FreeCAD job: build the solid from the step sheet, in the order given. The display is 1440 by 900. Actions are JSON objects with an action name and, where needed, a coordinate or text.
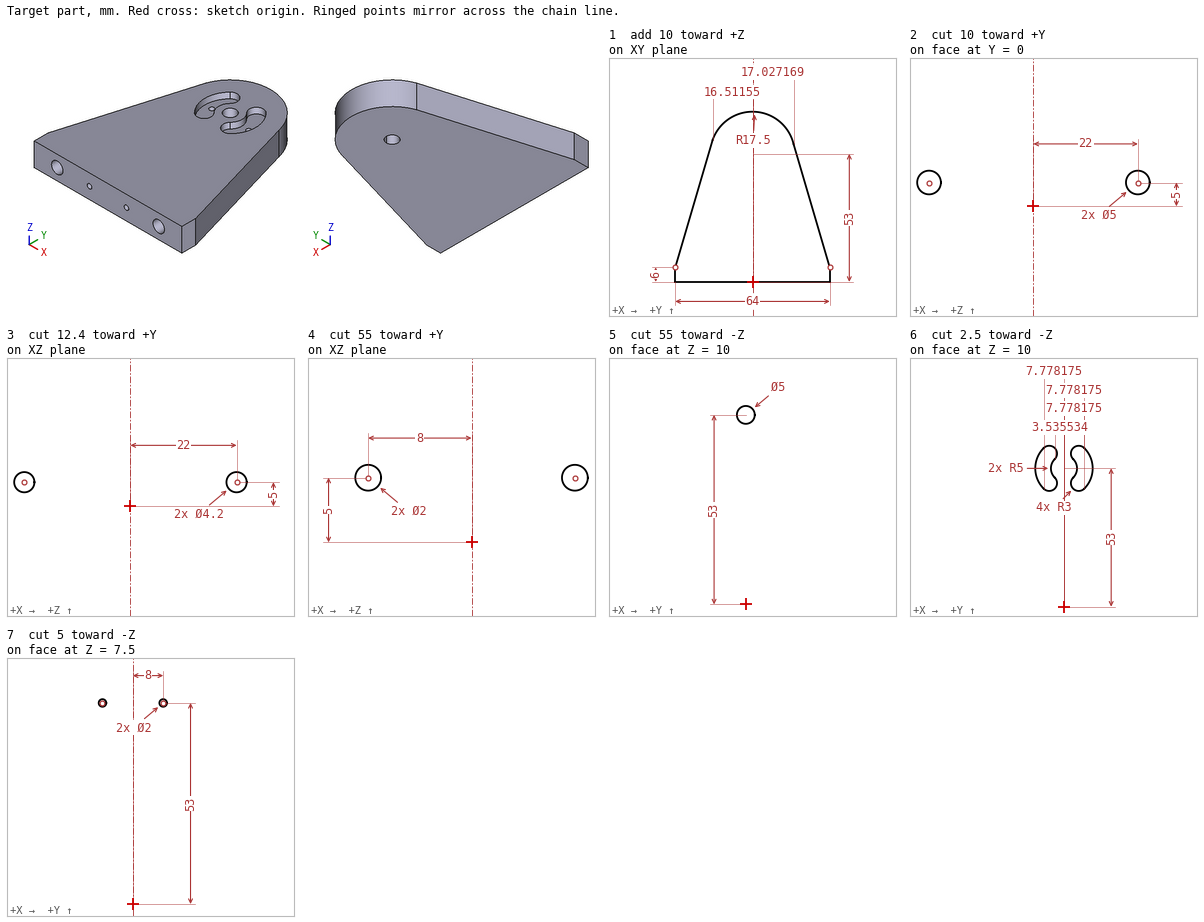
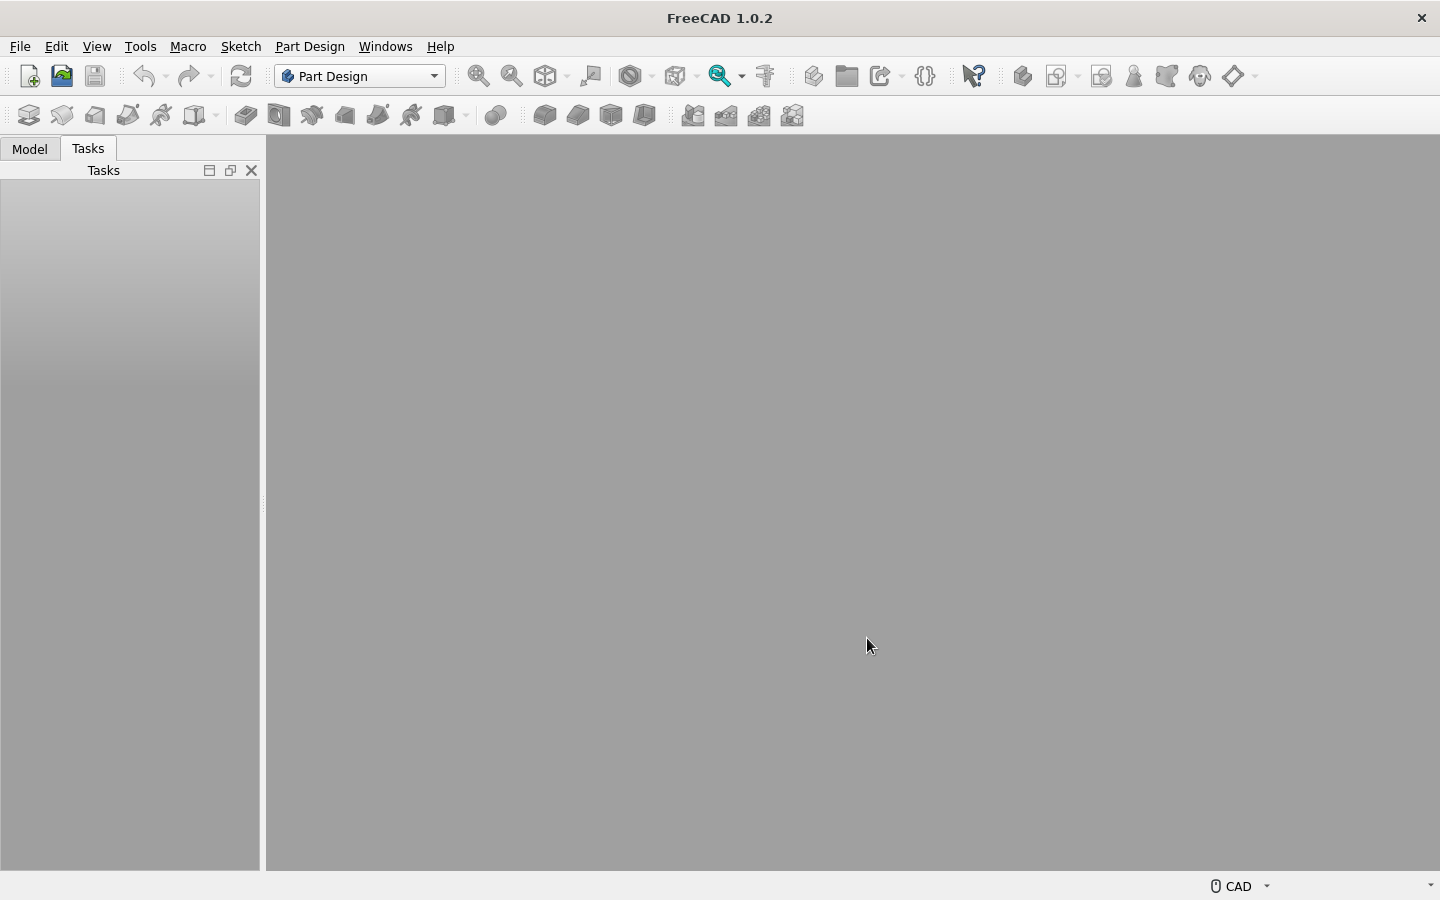
{"action": "left_click", "coordinate": [29, 76]}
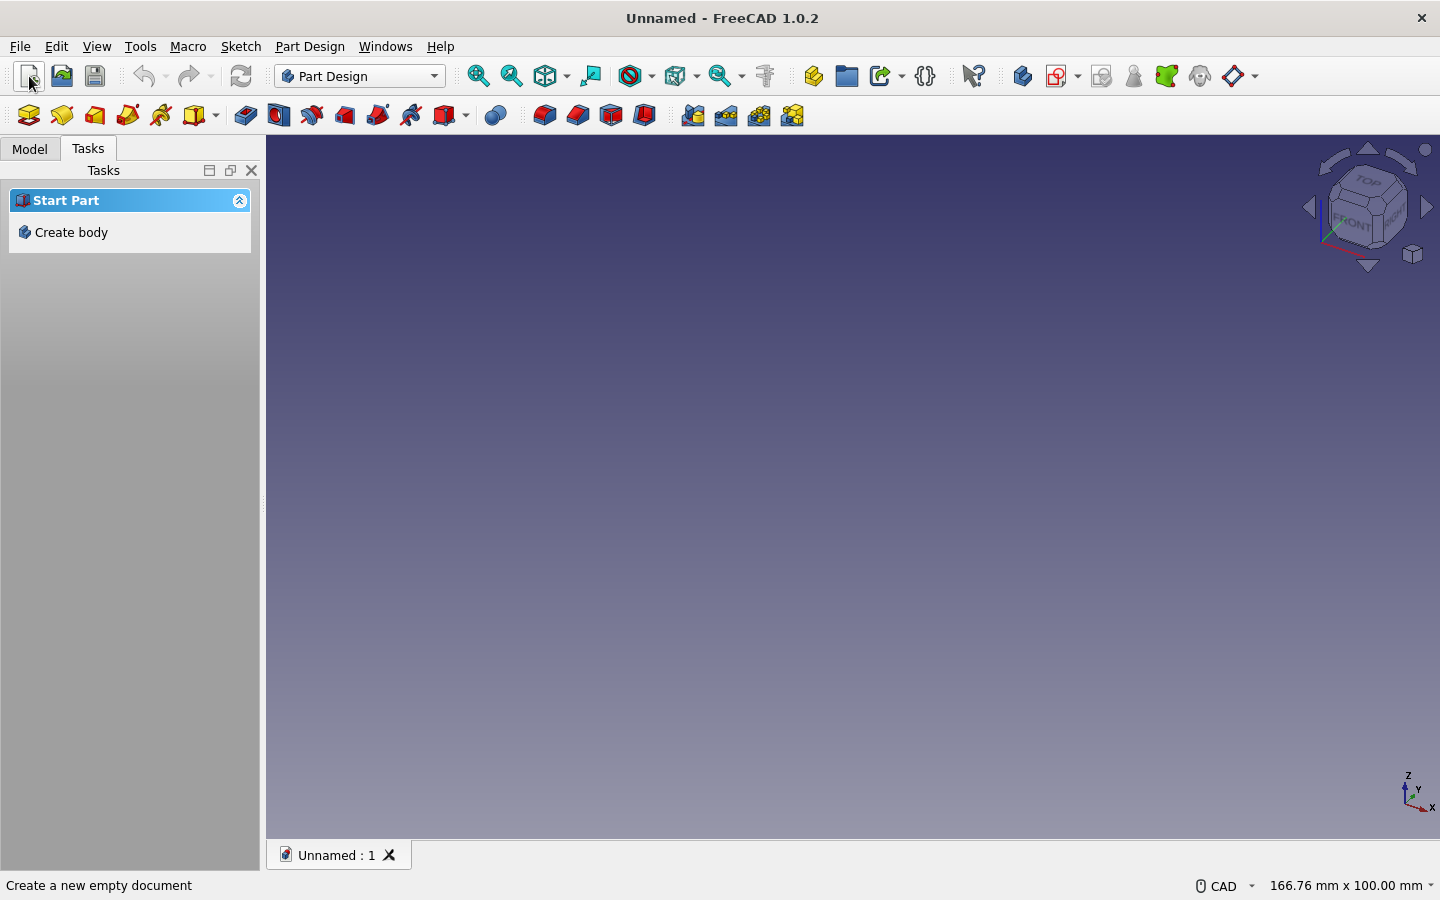
{"action": "left_click", "coordinate": [1056, 76]}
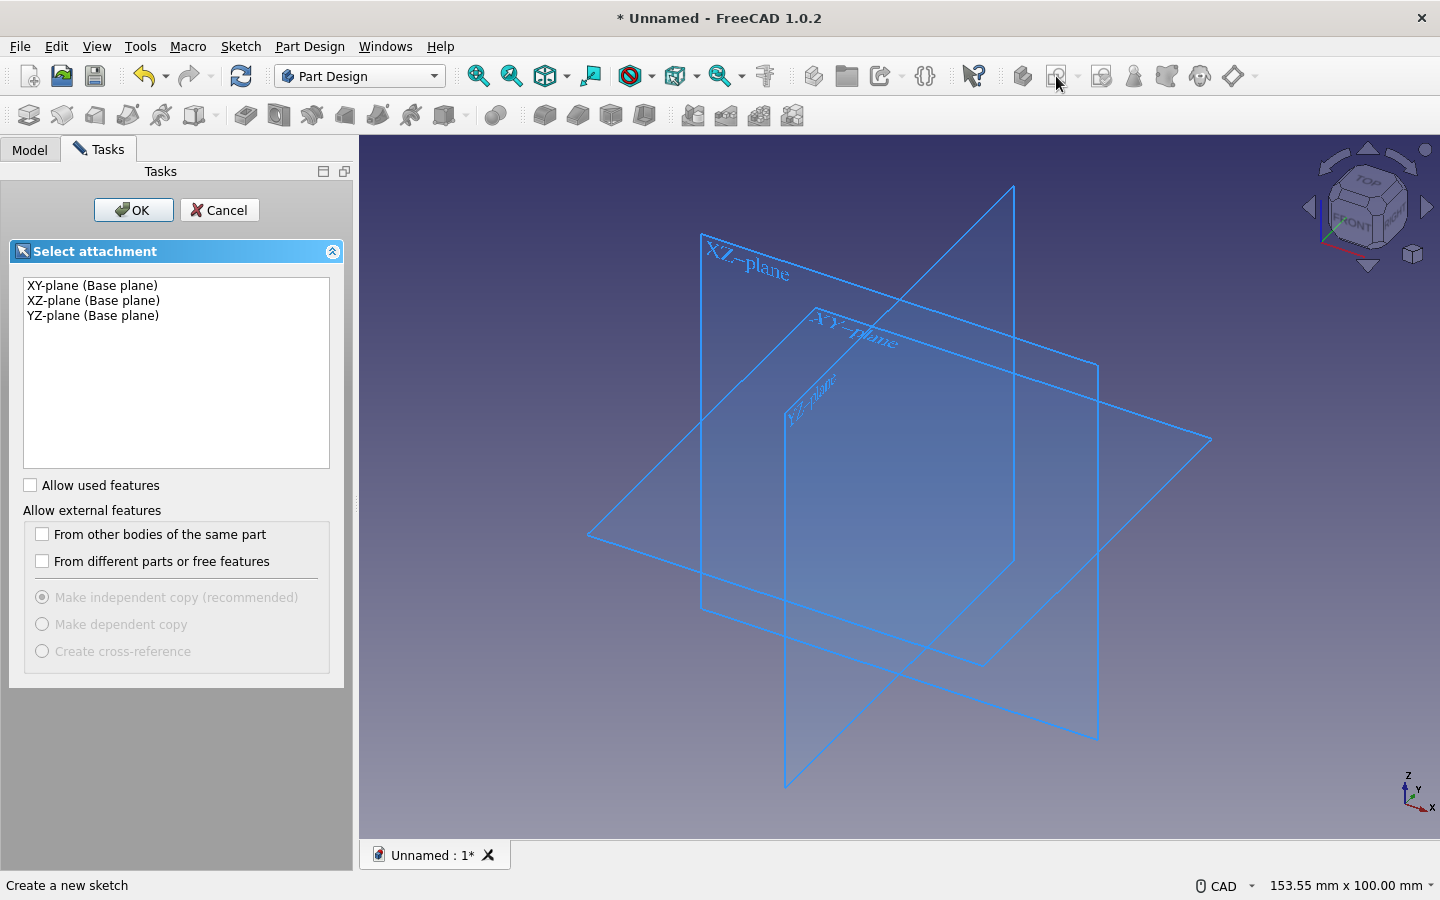
{"action": "left_click", "coordinate": [84, 286]}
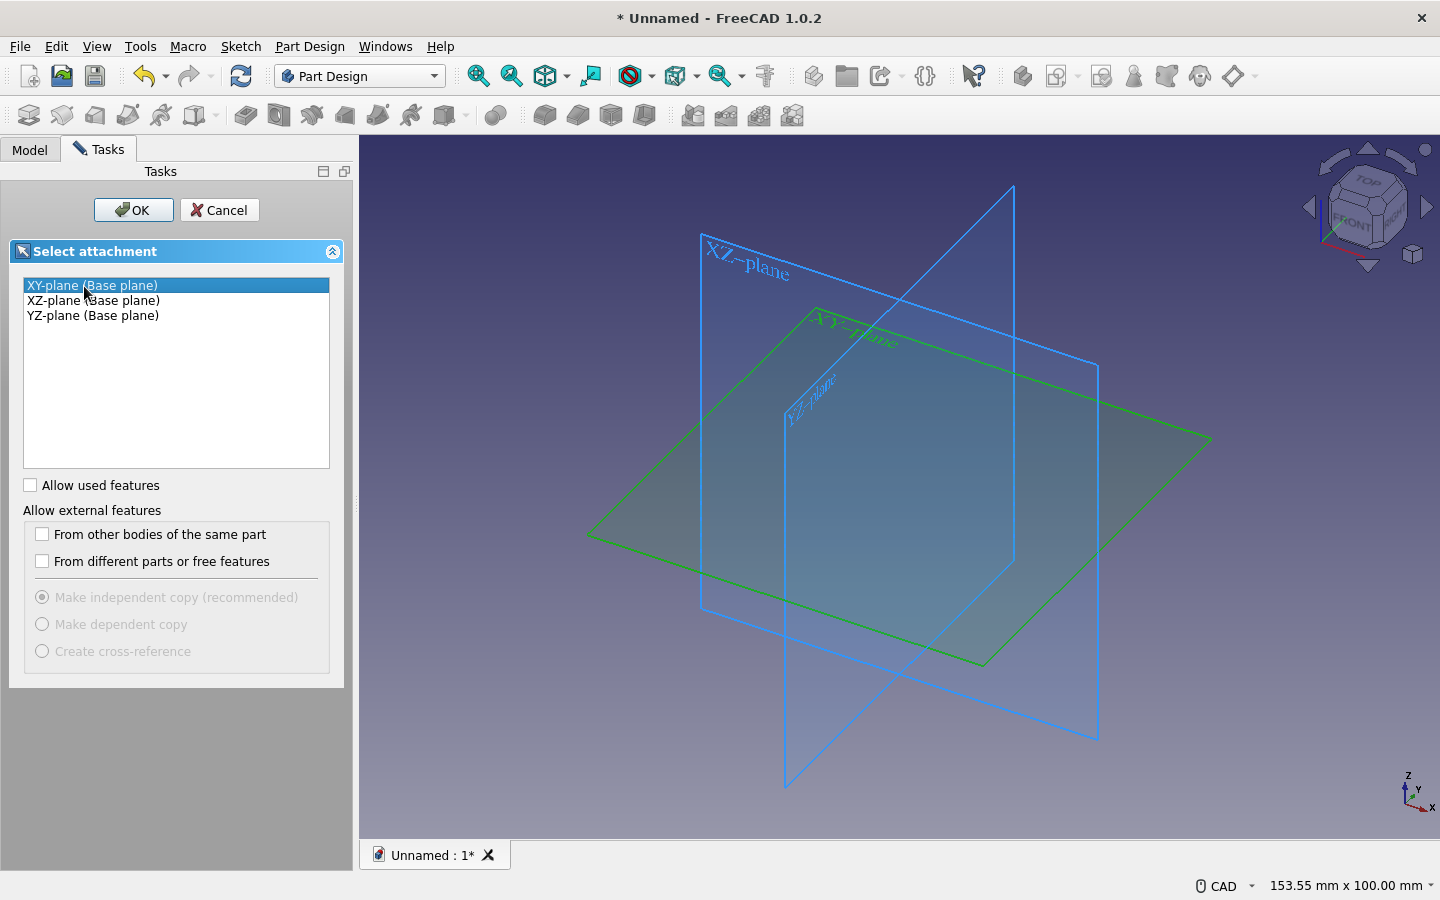
{"action": "left_click", "coordinate": [134, 210]}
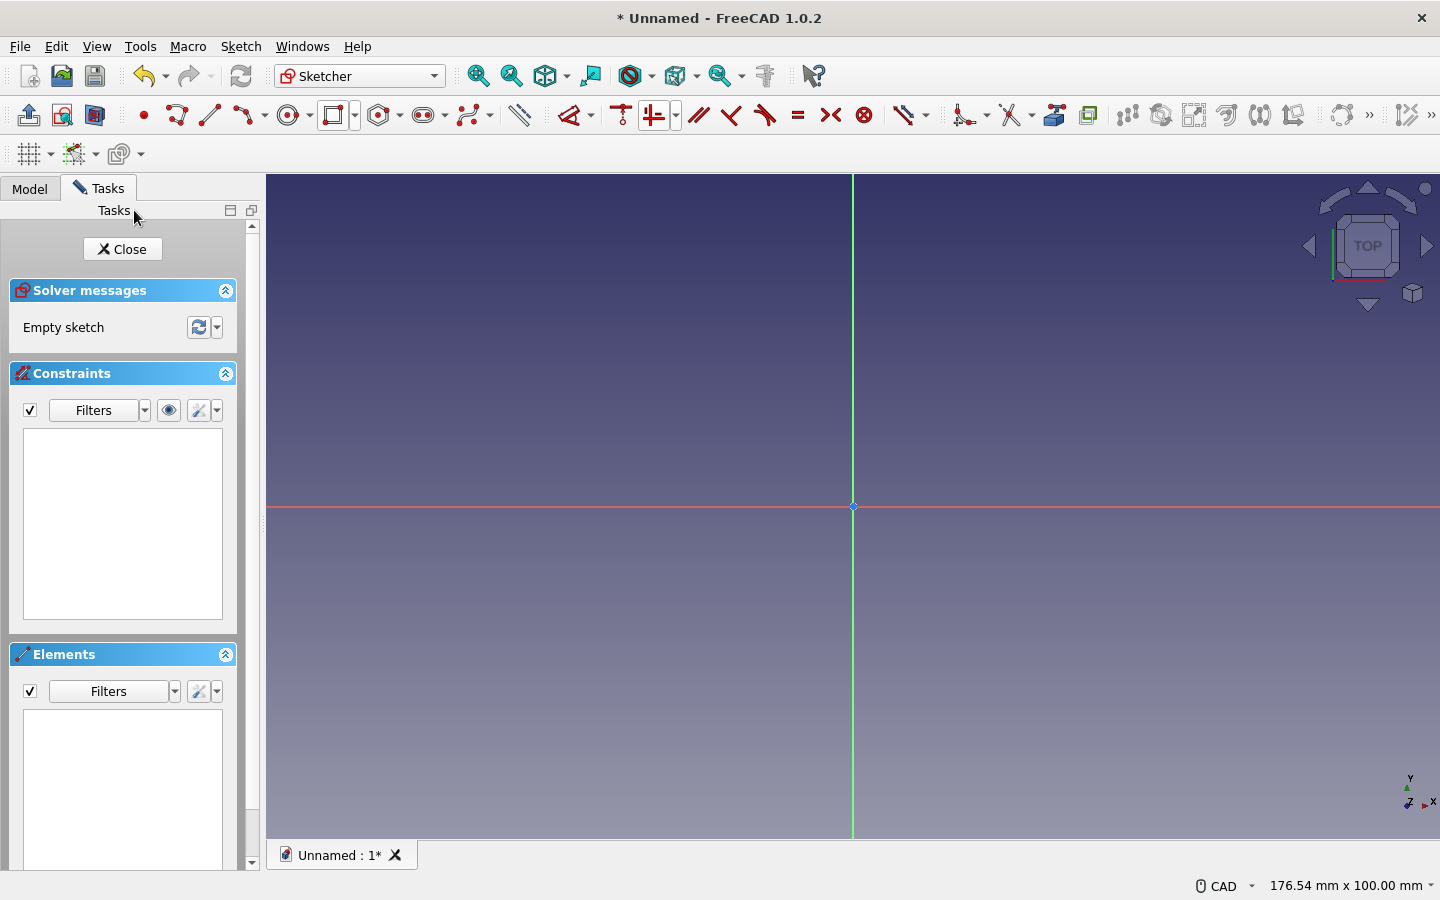
{"action": "scroll", "coordinate": [645, 811], "scroll_direction": "down", "scroll_amount": 2}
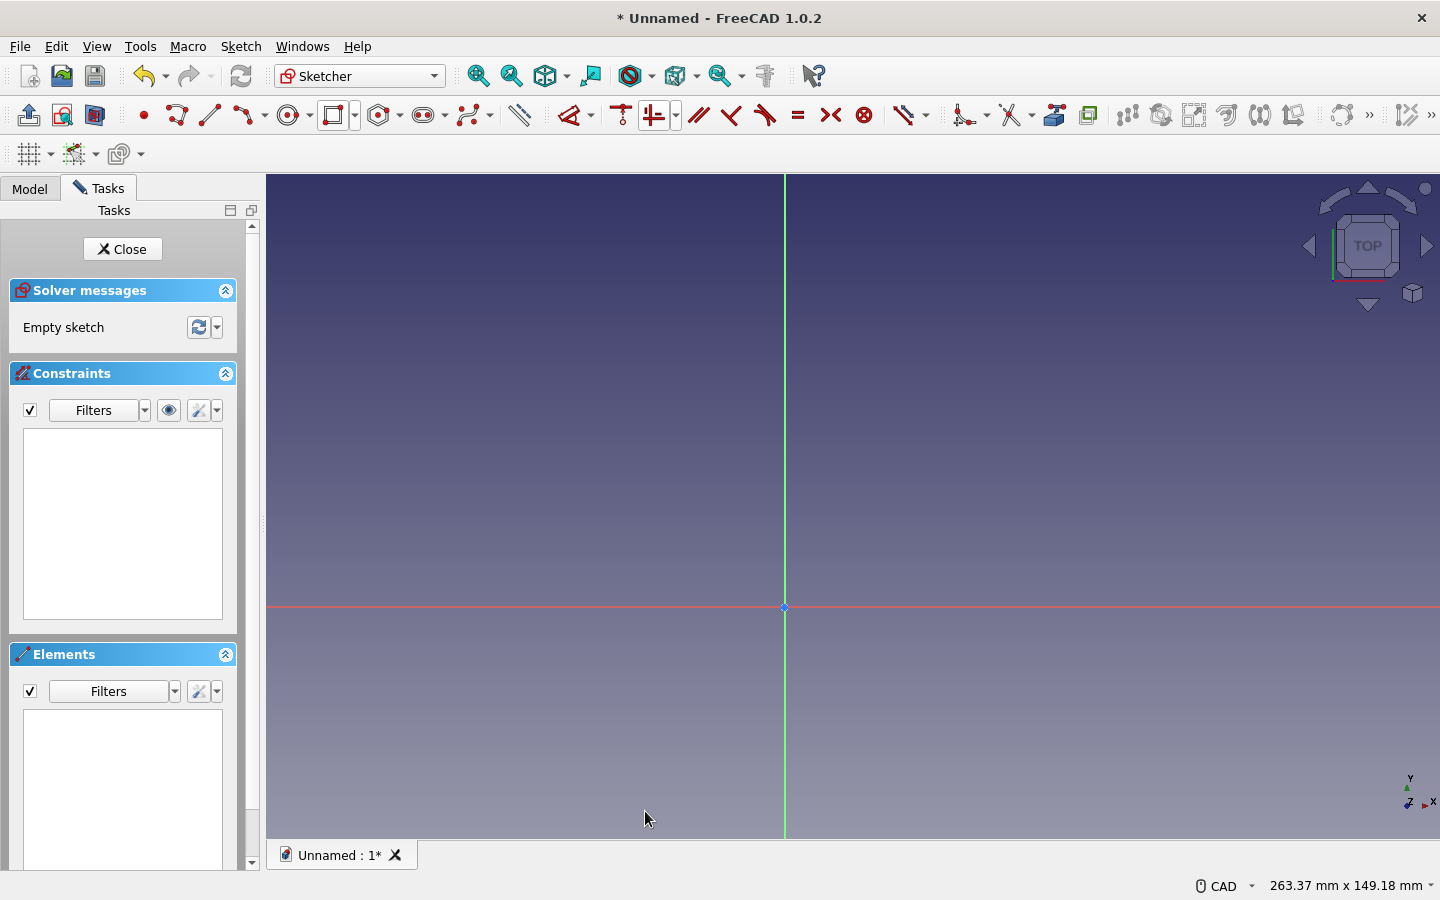
{"action": "scroll", "coordinate": [785, 336], "scroll_direction": "up", "scroll_amount": 2}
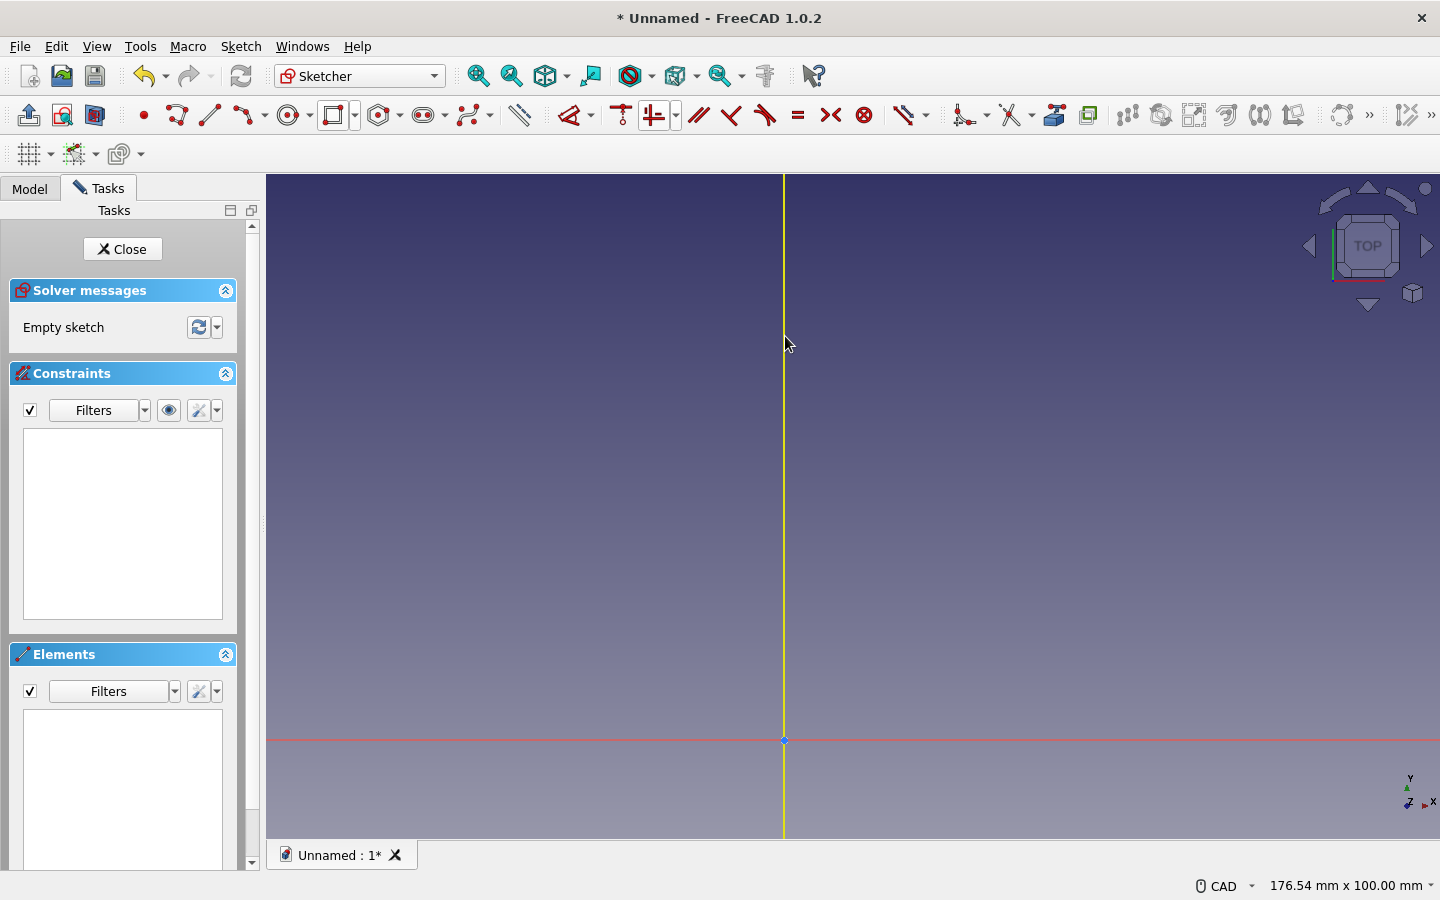
{"action": "left_click", "coordinate": [177, 116]}